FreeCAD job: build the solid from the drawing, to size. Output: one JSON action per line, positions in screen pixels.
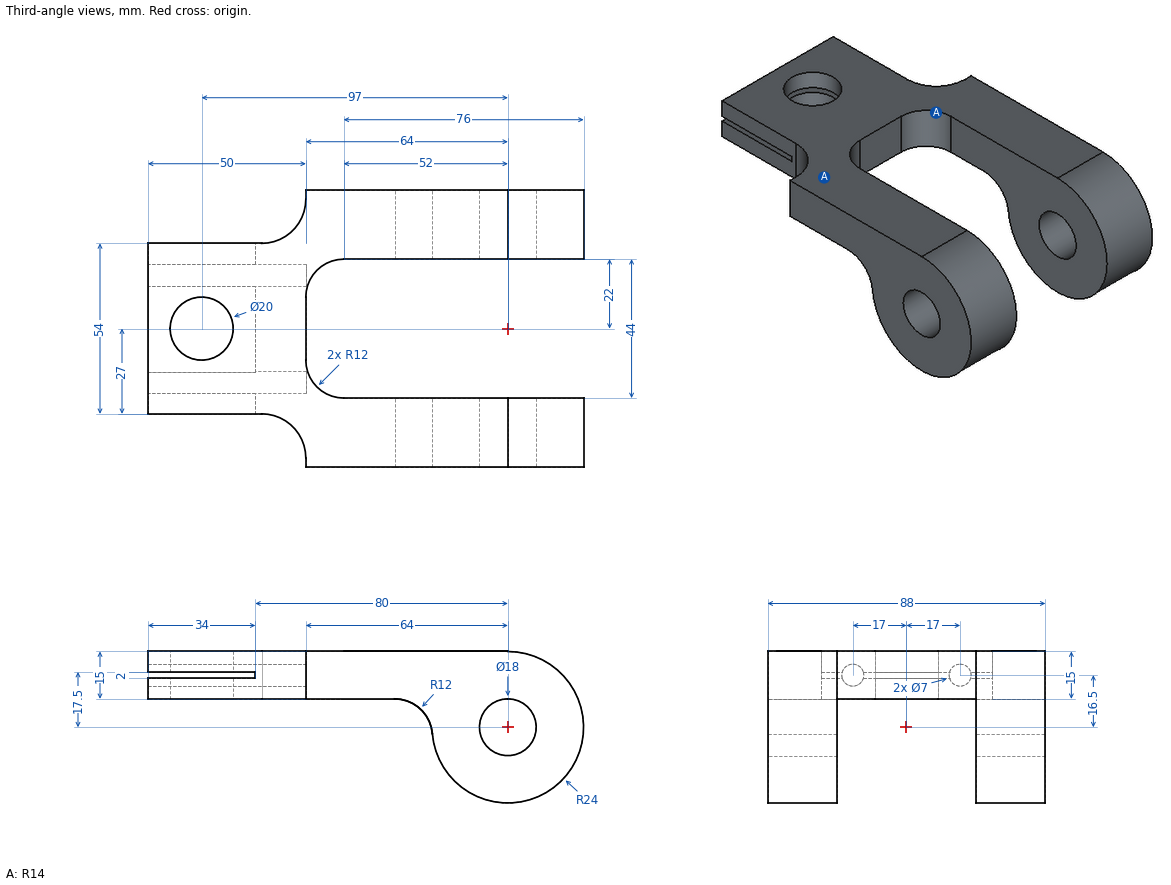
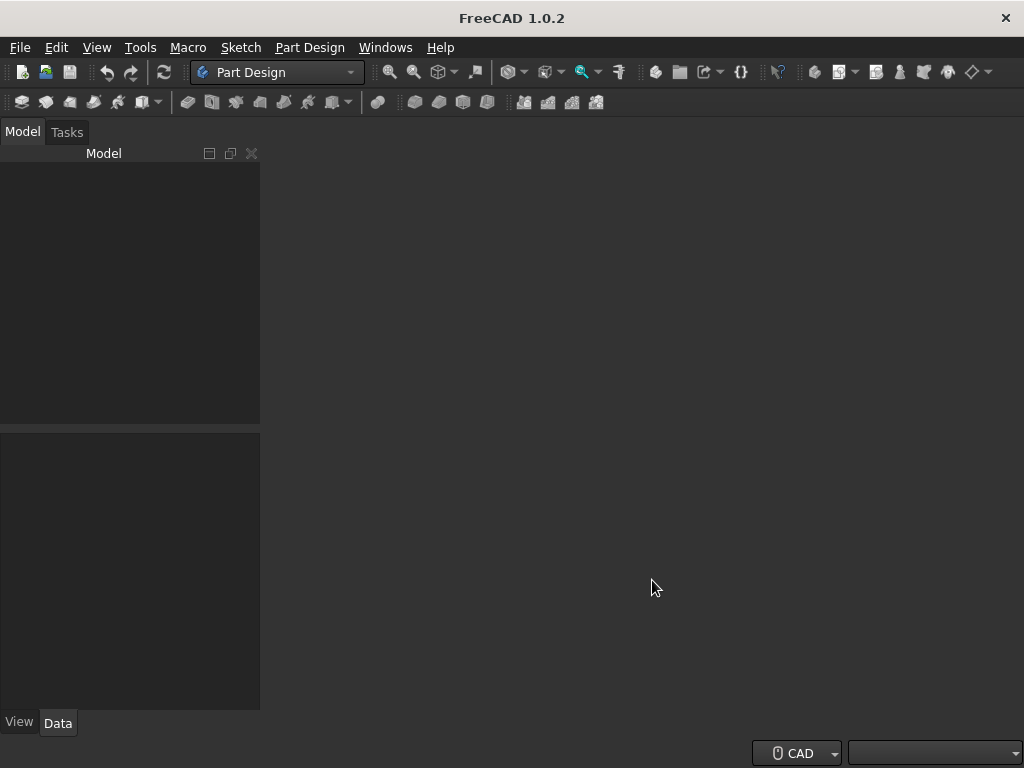
{"action": "left_click", "coordinate": [22, 72]}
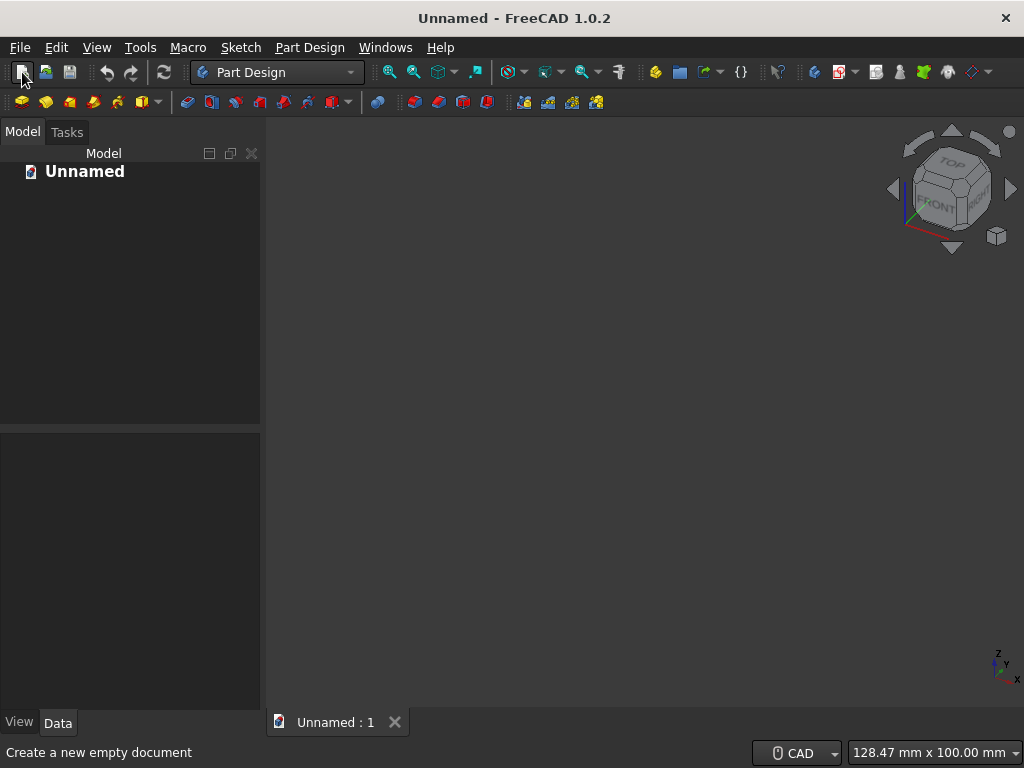
{"action": "left_click", "coordinate": [840, 72]}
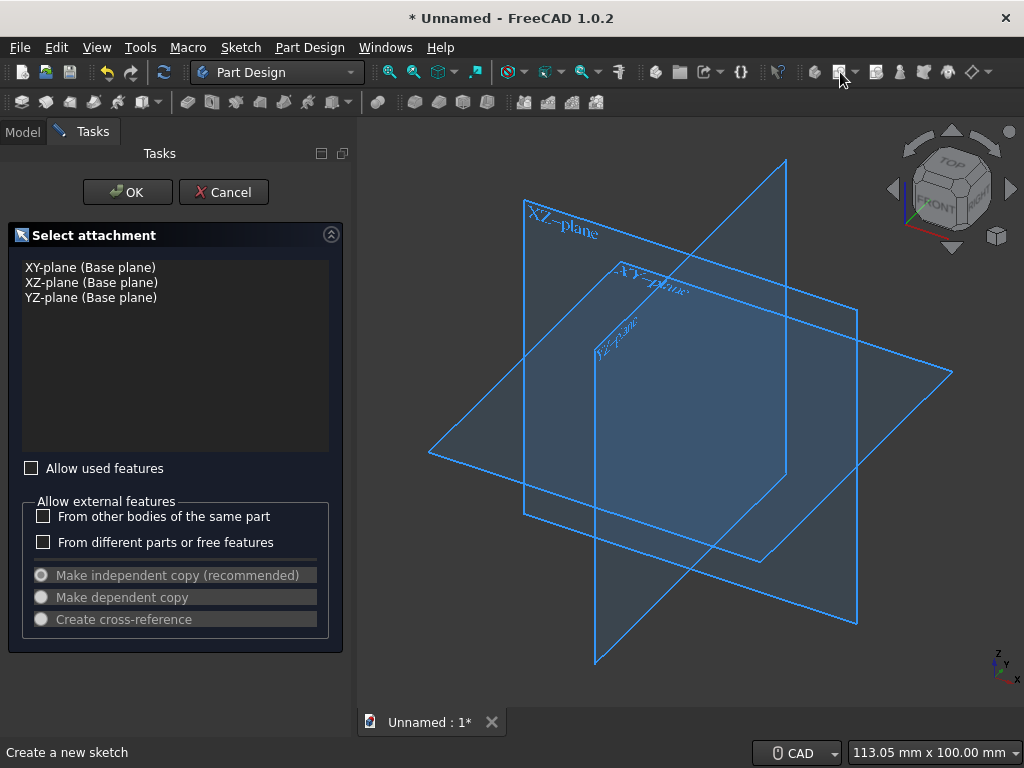
{"action": "left_click", "coordinate": [82, 282]}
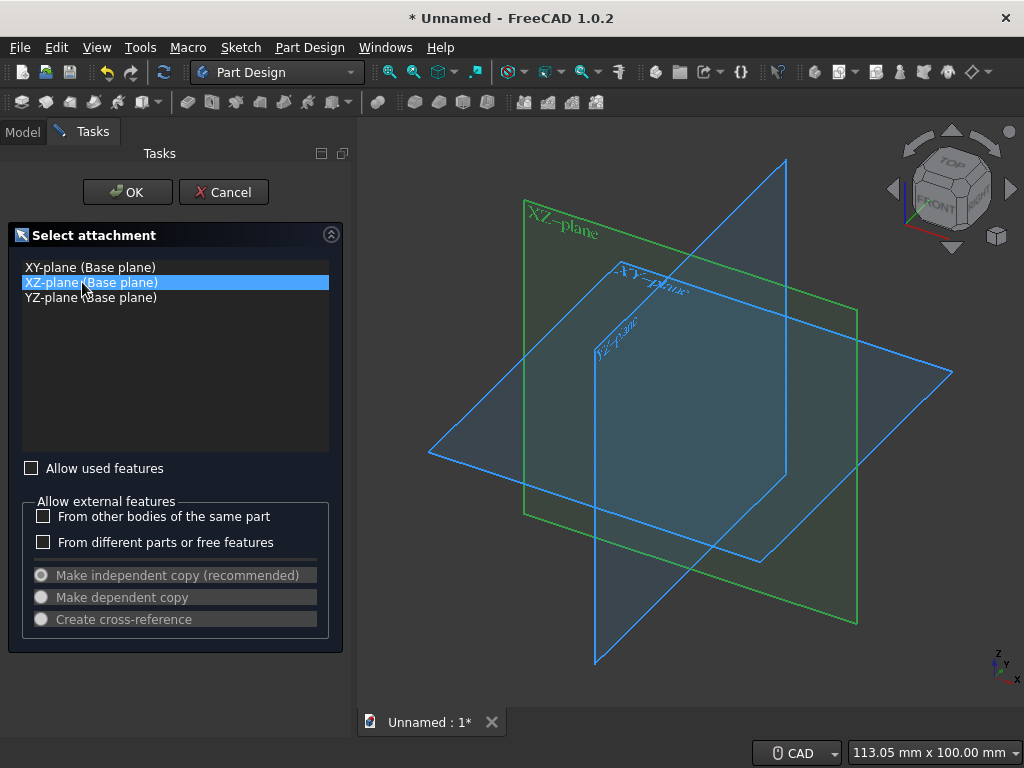
{"action": "left_click", "coordinate": [128, 192]}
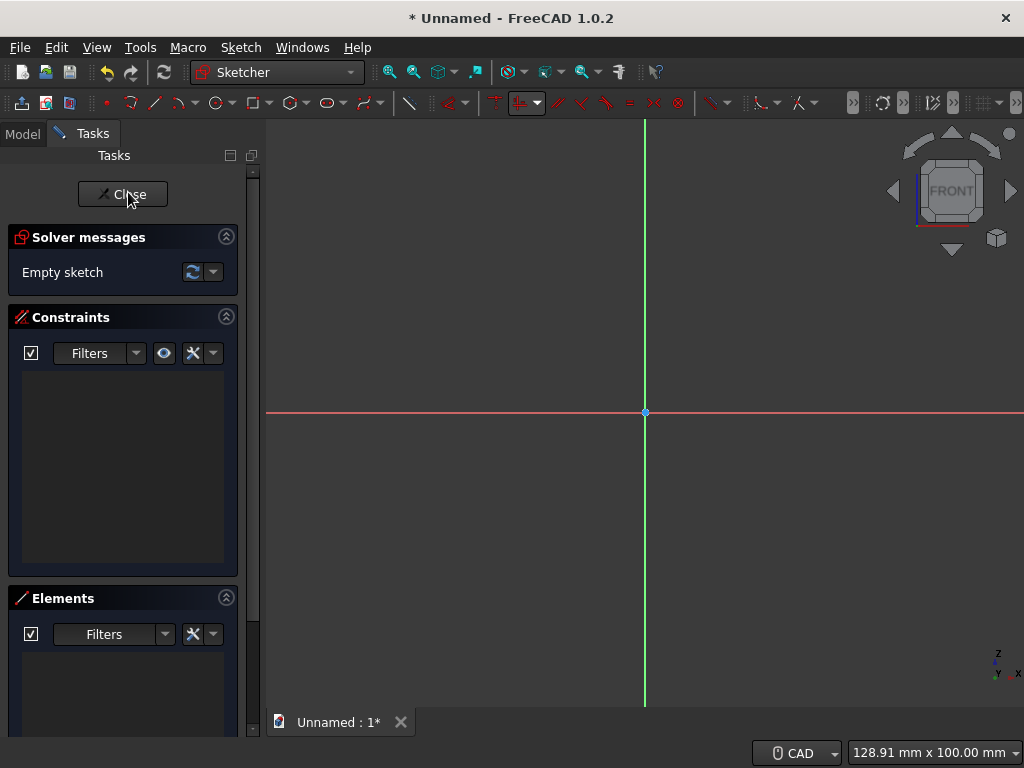
{"action": "scroll", "coordinate": [859, 516], "scroll_direction": "down", "scroll_amount": 1}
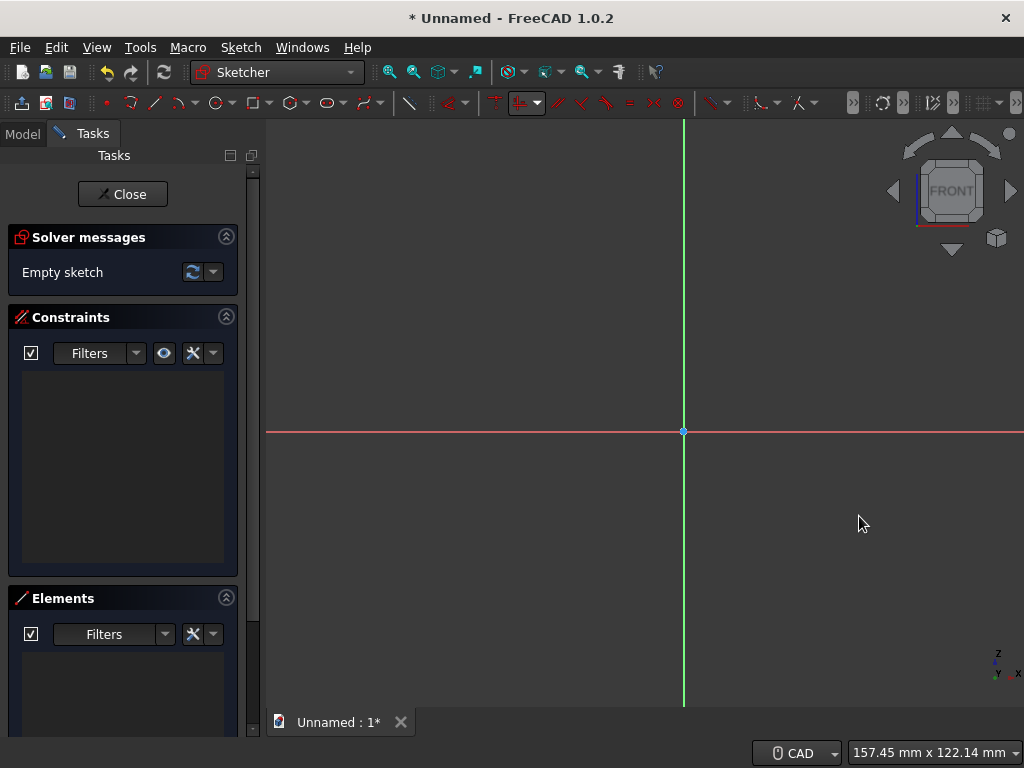
{"action": "left_click", "coordinate": [132, 104]}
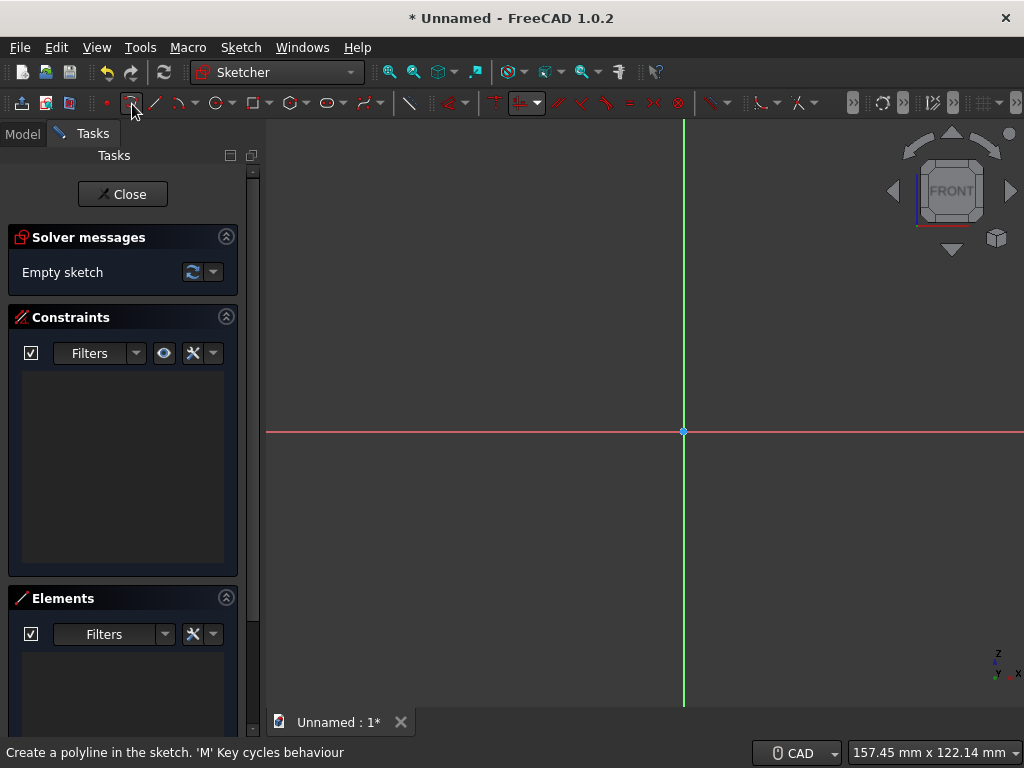
{"action": "left_click", "coordinate": [511, 388]}
{"action": "left_click", "coordinate": [376, 388]}
{"action": "left_click", "coordinate": [376, 316]}
{"action": "left_click", "coordinate": [684, 316]}
{"action": "right_click", "coordinate": [684, 316]}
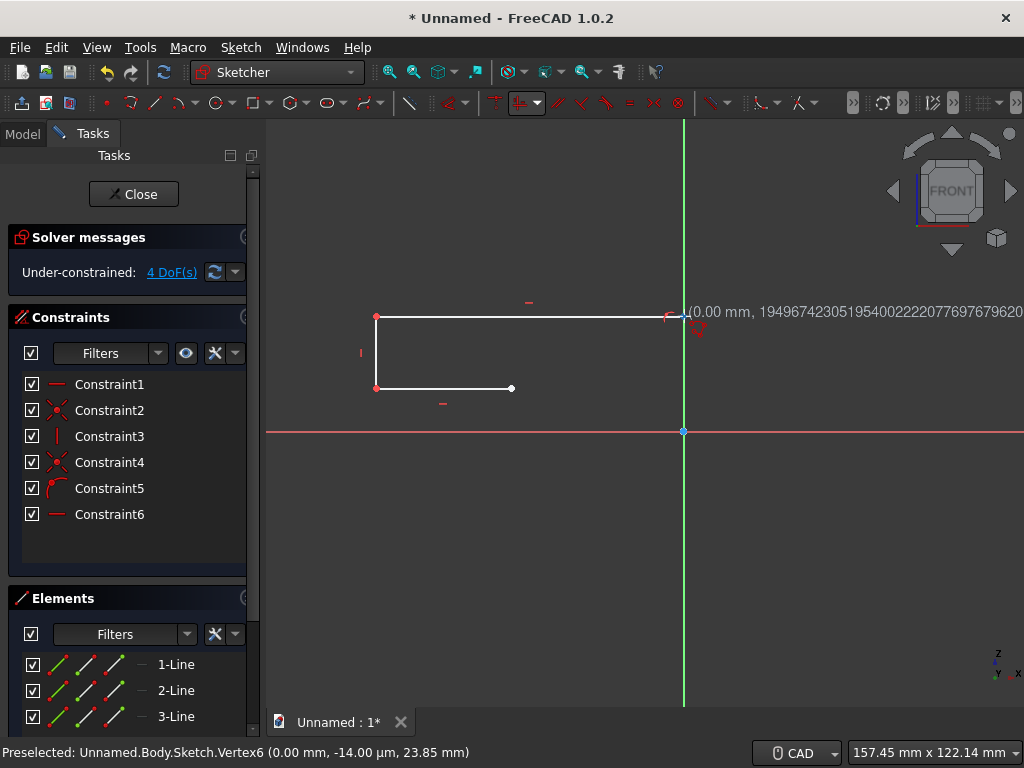
{"action": "key", "text": "g 3 a"}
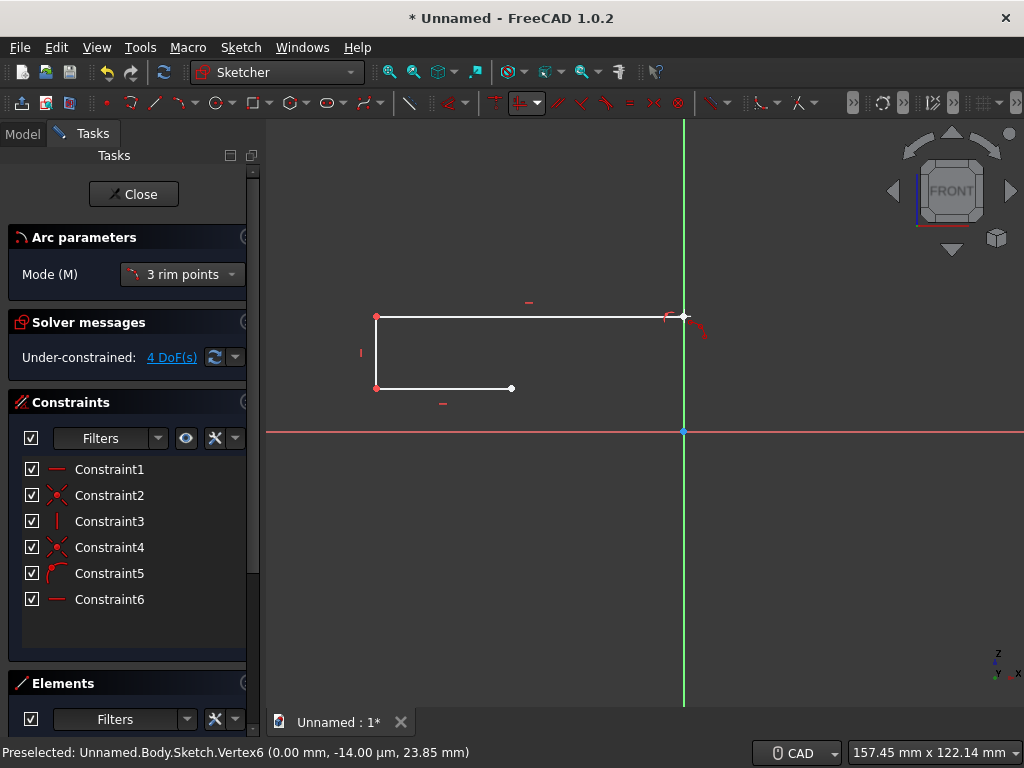
{"action": "left_click", "coordinate": [684, 317]}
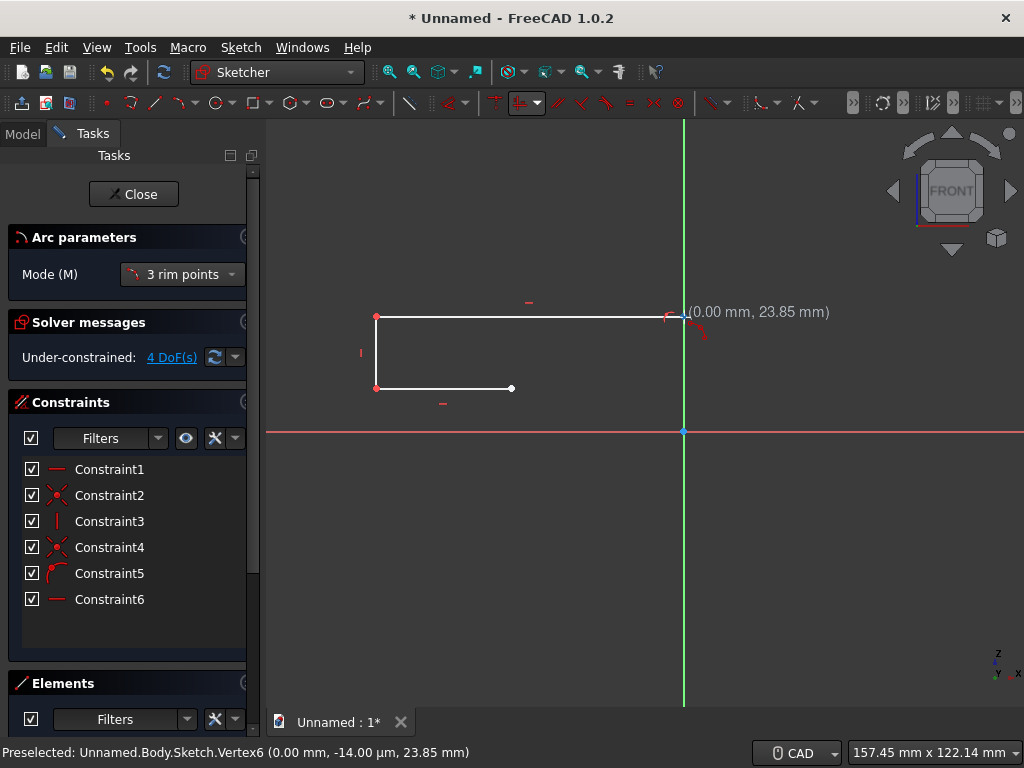
{"action": "scroll", "coordinate": [569, 441], "scroll_direction": "up", "scroll_amount": 3}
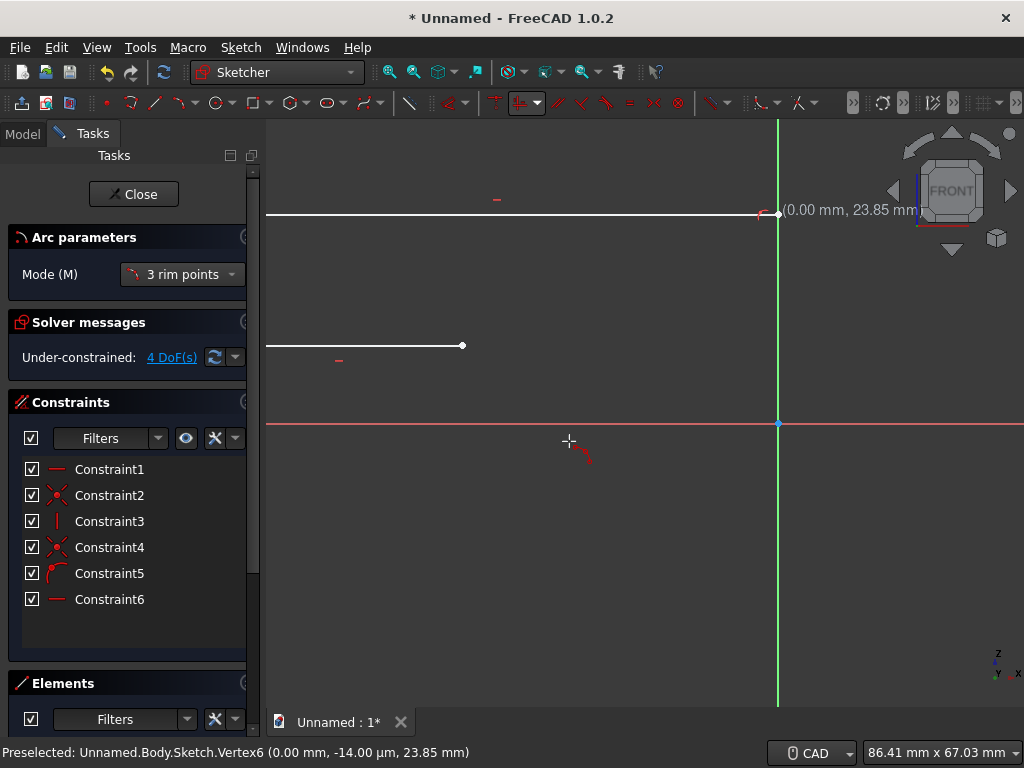
{"action": "left_click", "coordinate": [568, 441]}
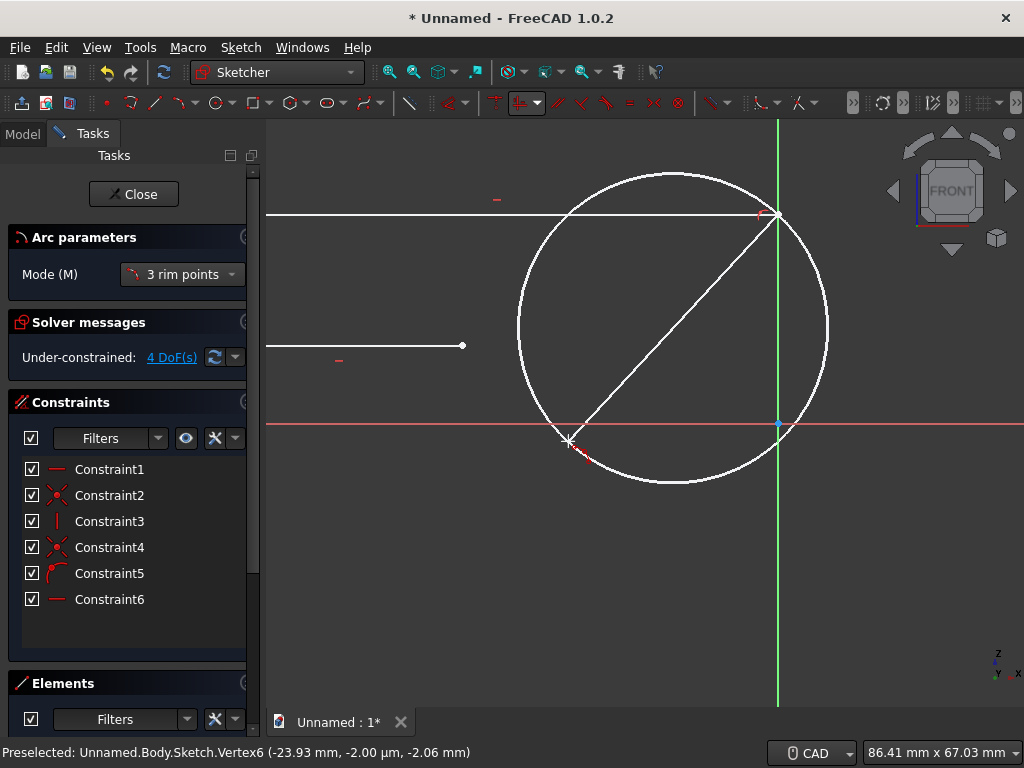
{"action": "scroll", "coordinate": [578, 441], "scroll_direction": "down", "scroll_amount": 3}